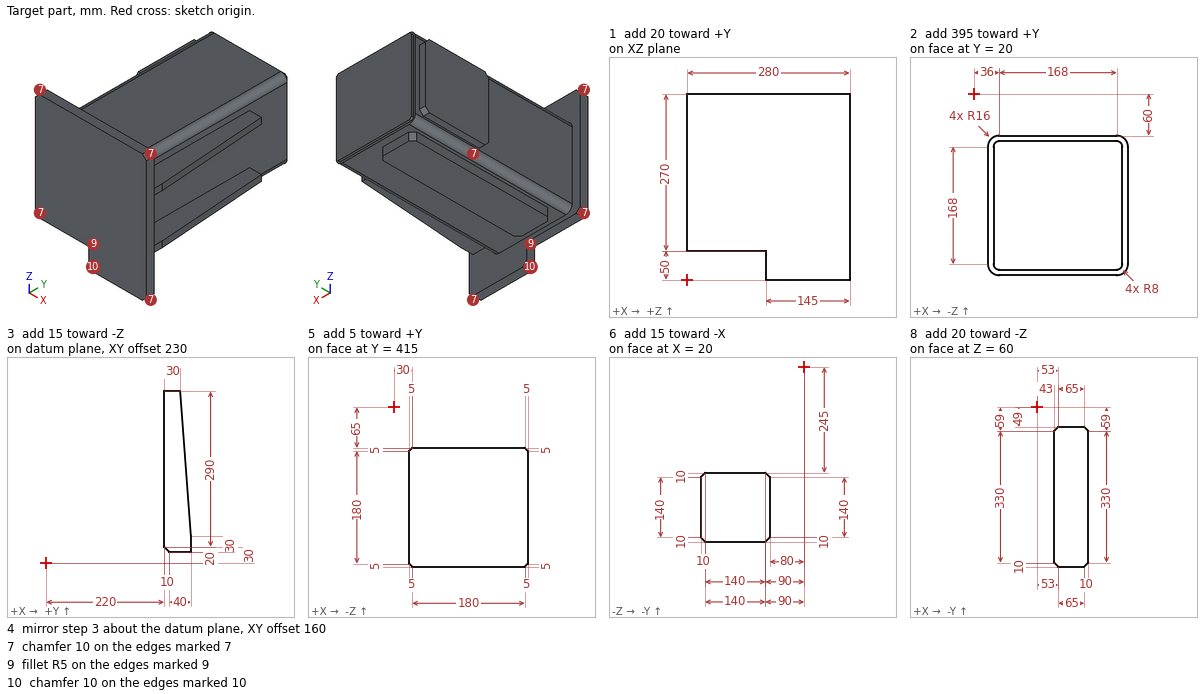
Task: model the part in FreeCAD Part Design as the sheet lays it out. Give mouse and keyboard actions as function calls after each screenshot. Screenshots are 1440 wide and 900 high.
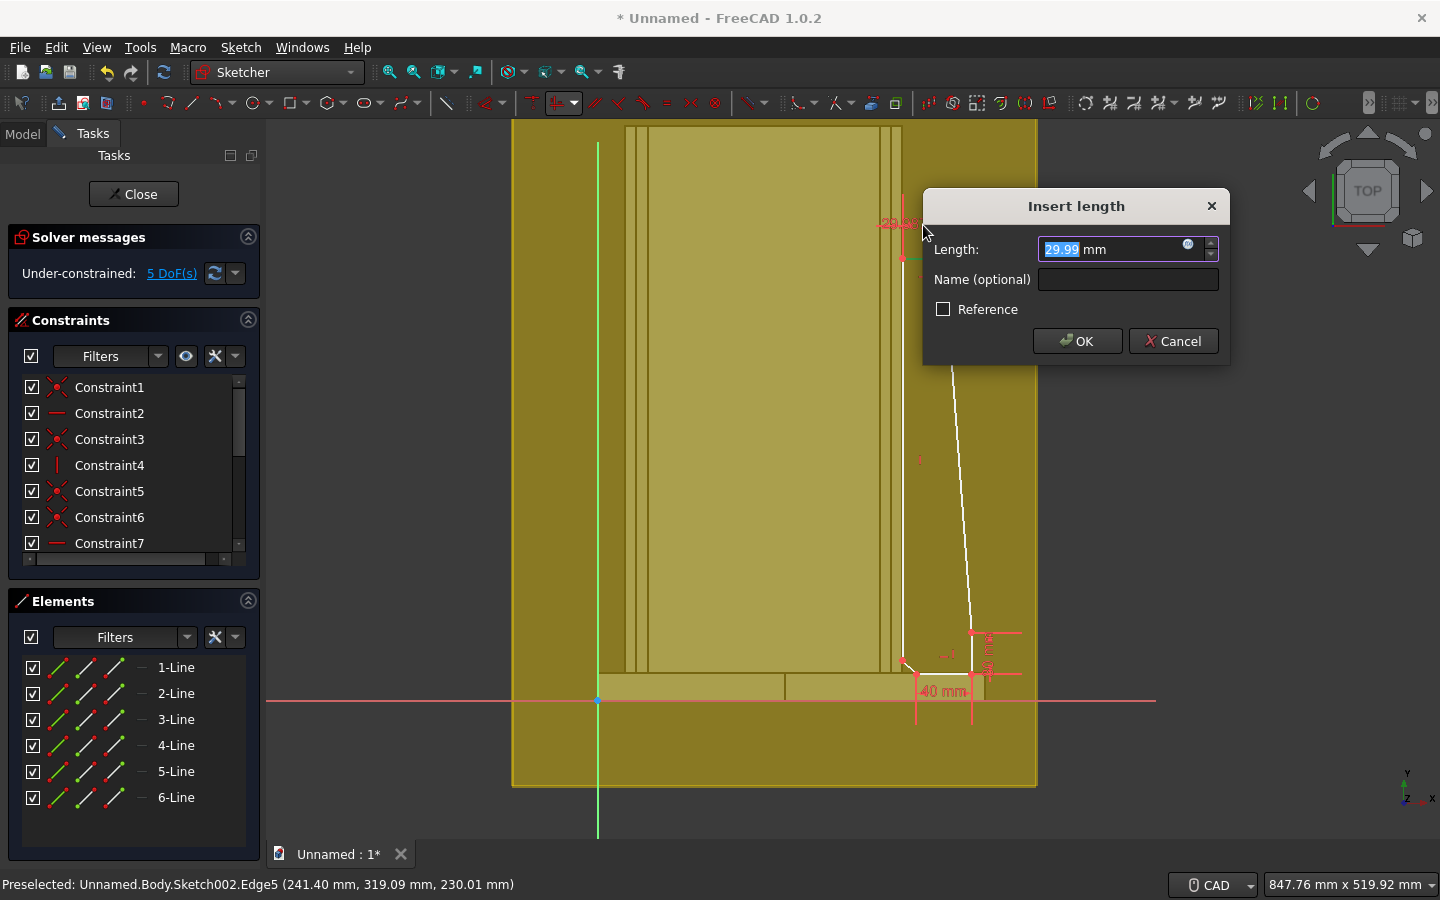
text(30)
key(Return)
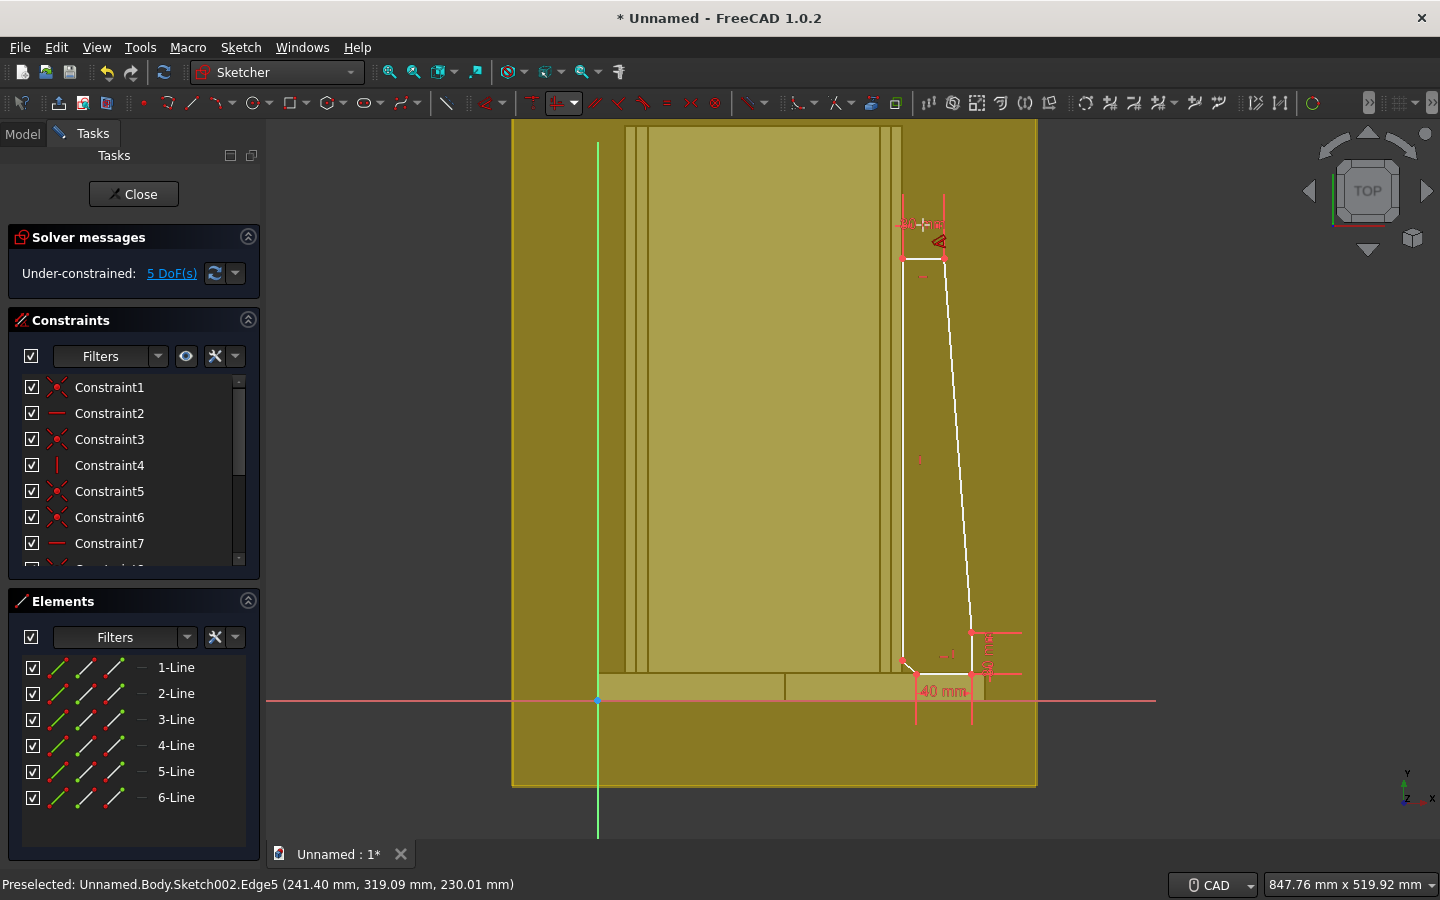
click(903, 379)
click(937, 460)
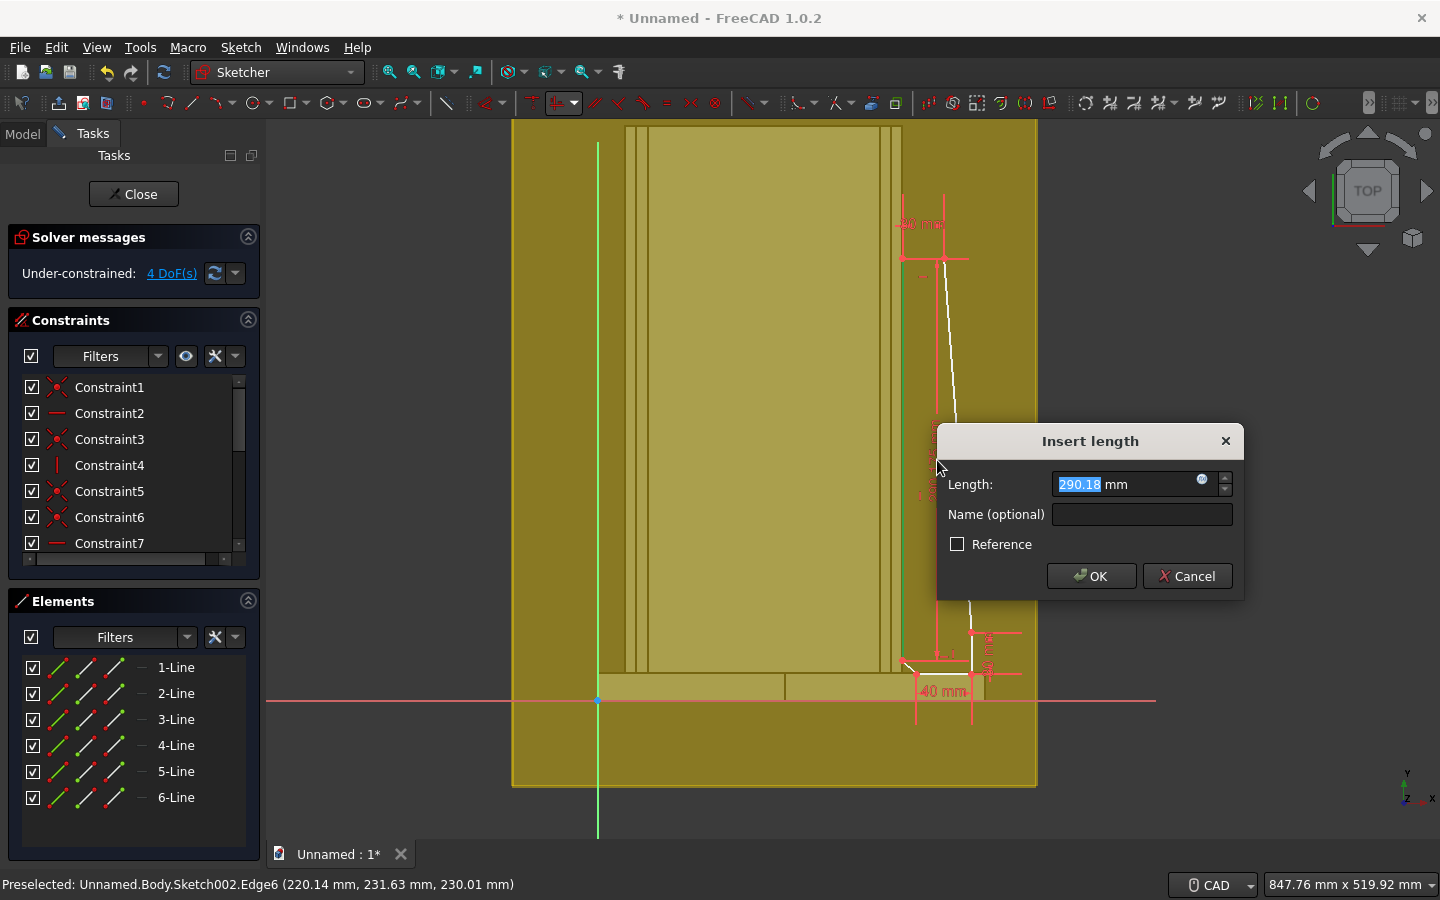
text(290)
key(Return)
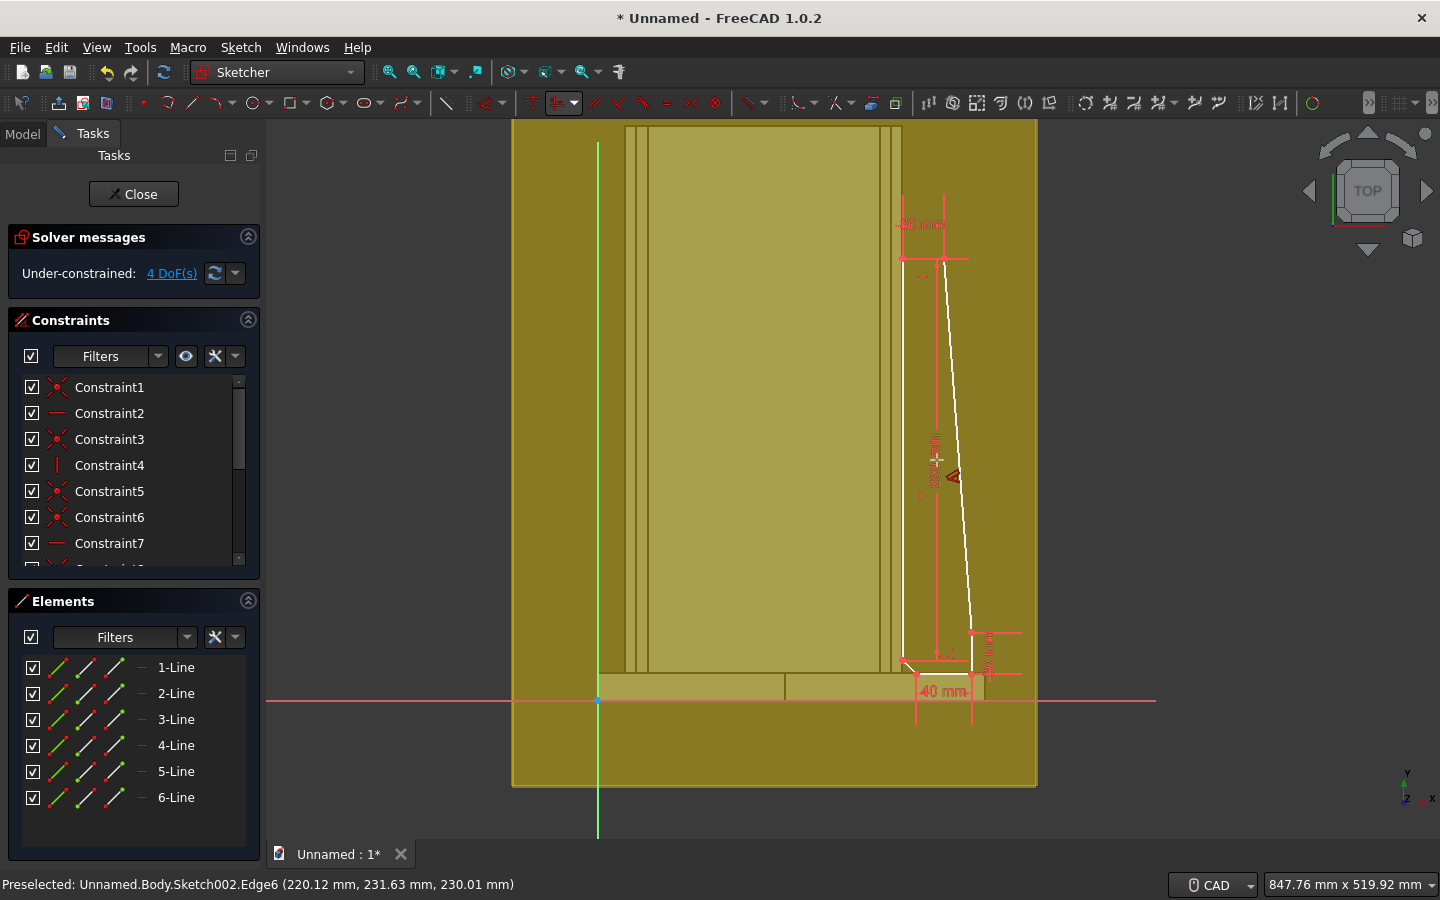
click(903, 661)
click(564, 681)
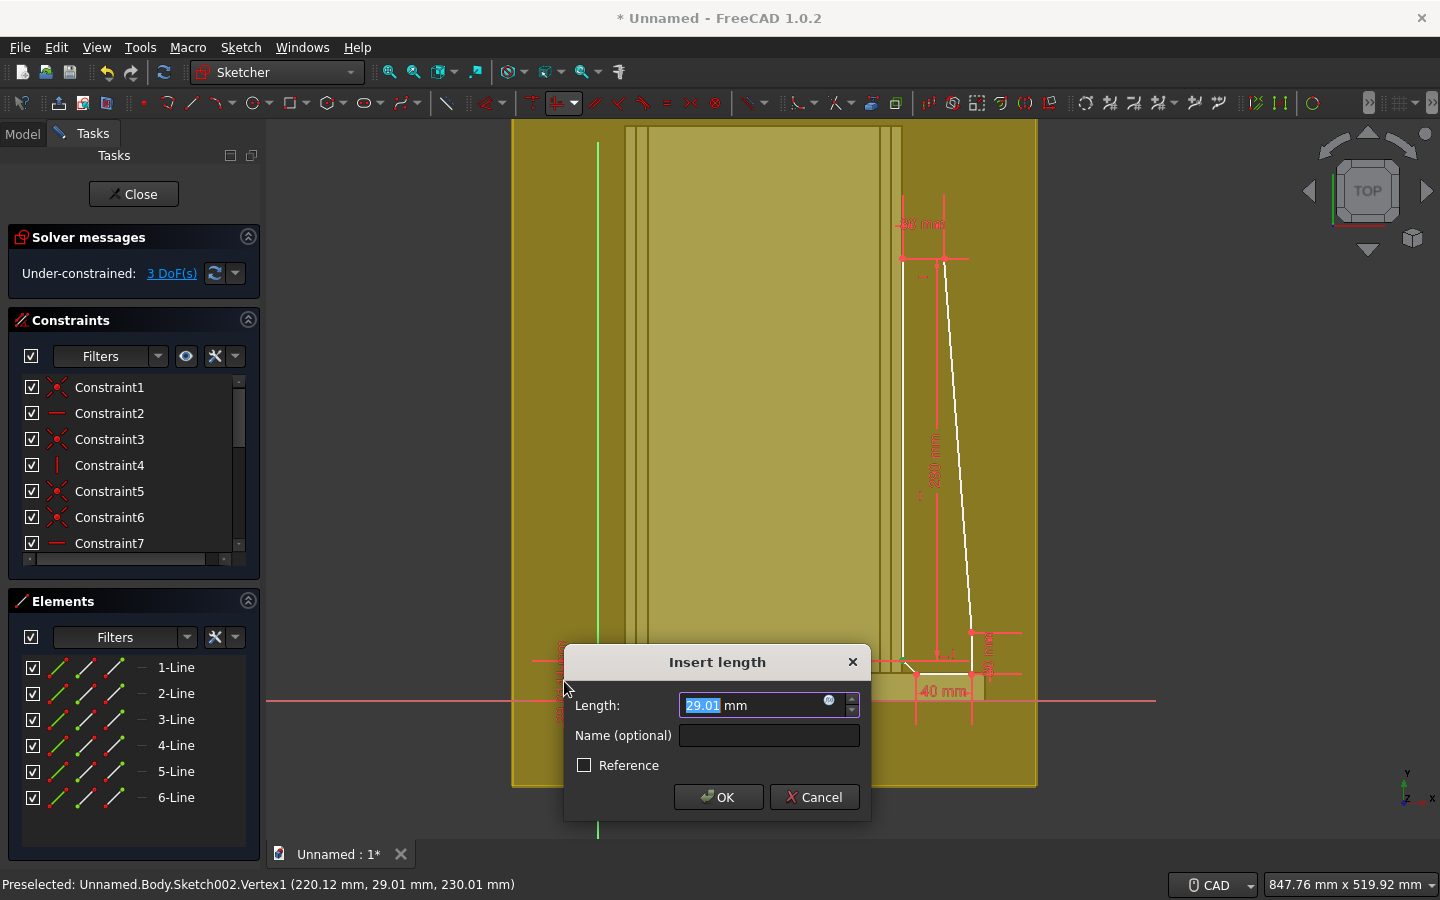
text(30)
key(Return)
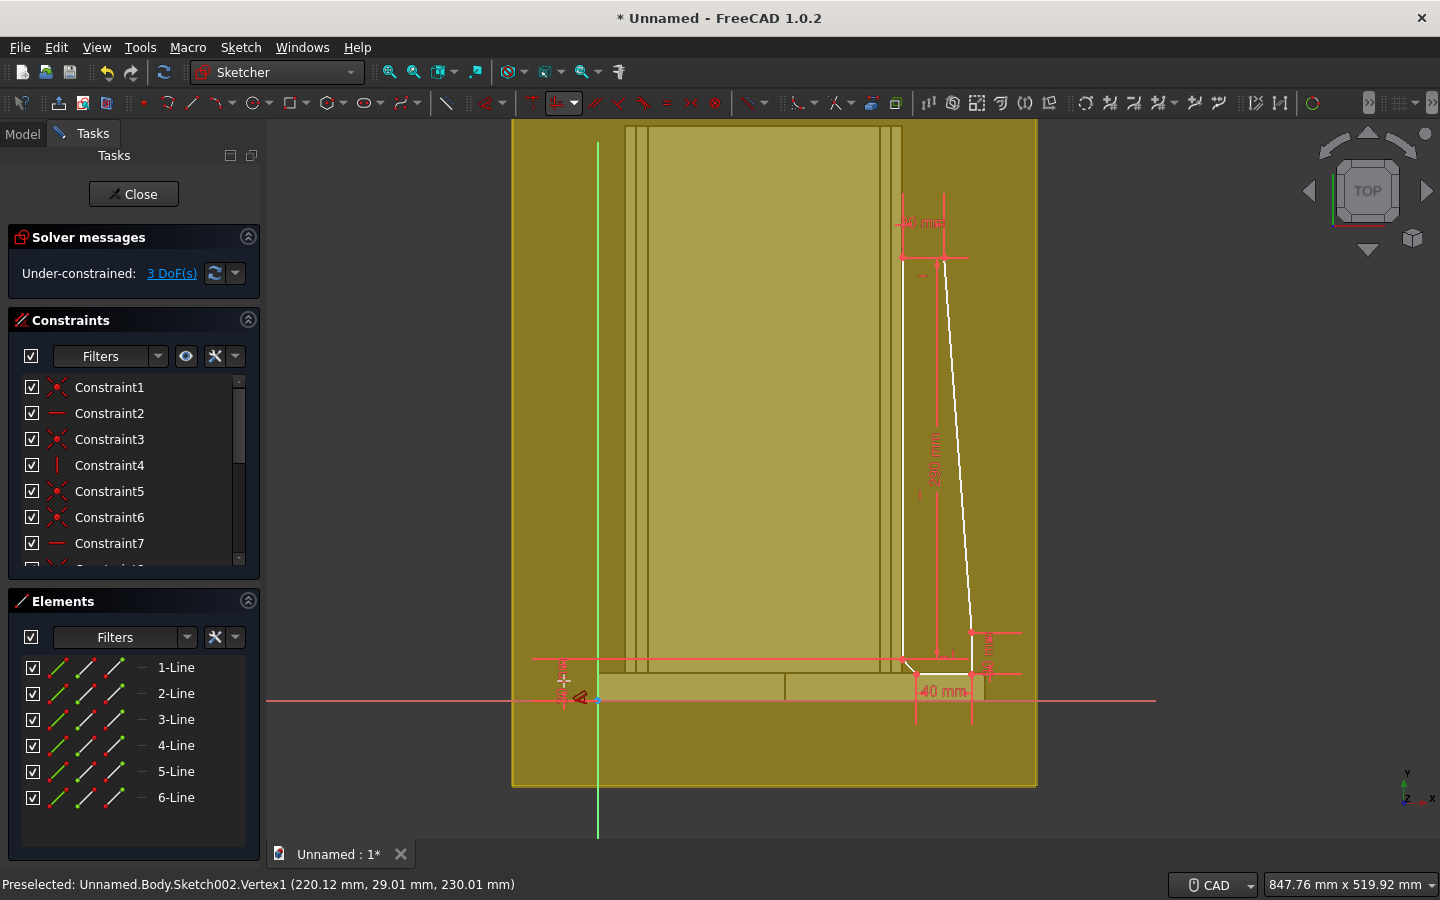
scroll(916, 674, up, 2)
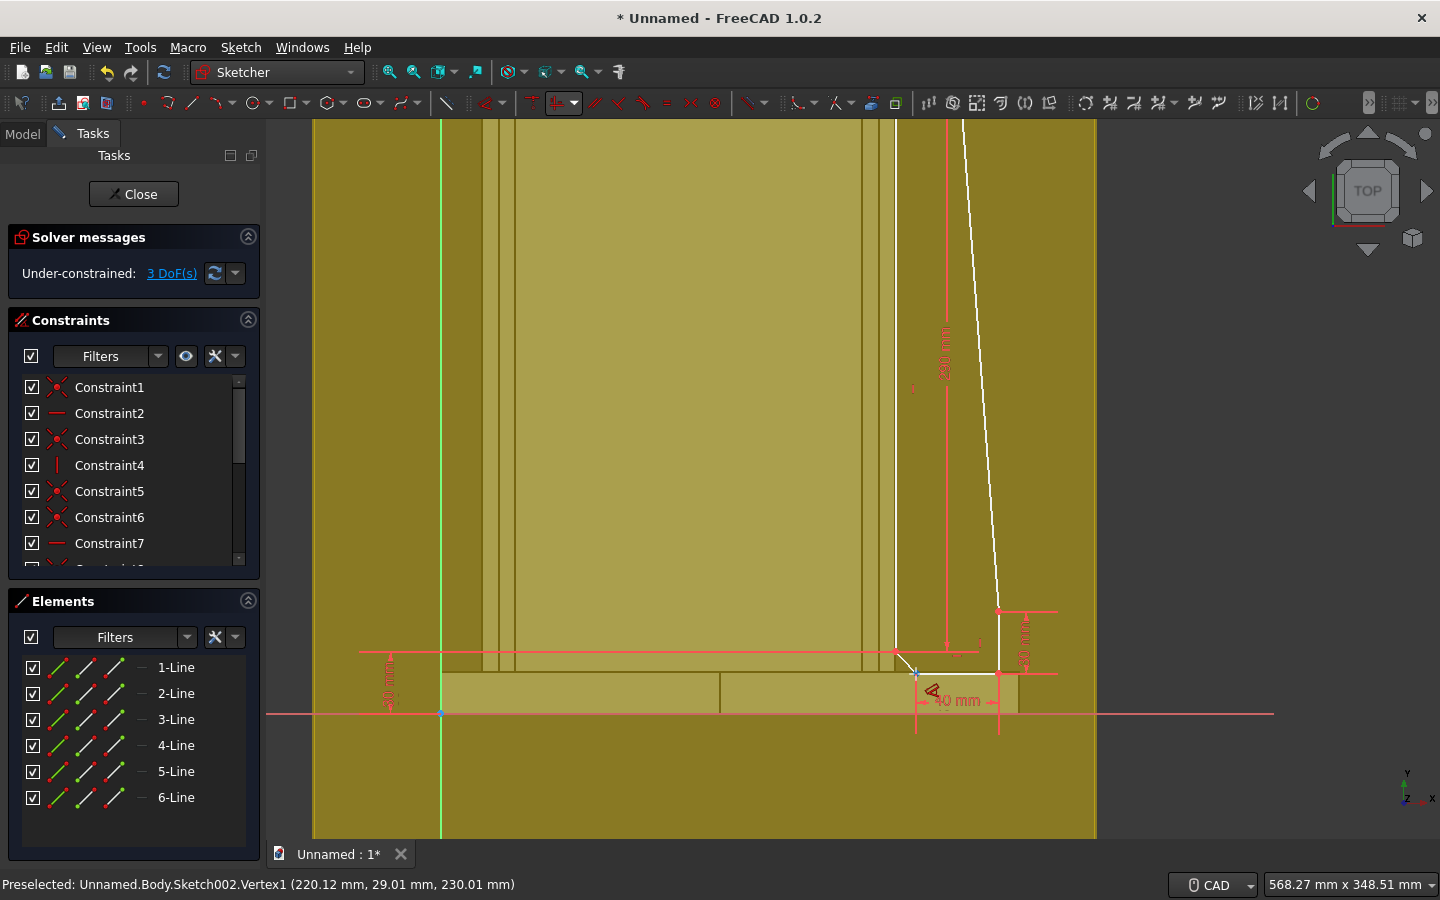
click(916, 674)
click(1022, 680)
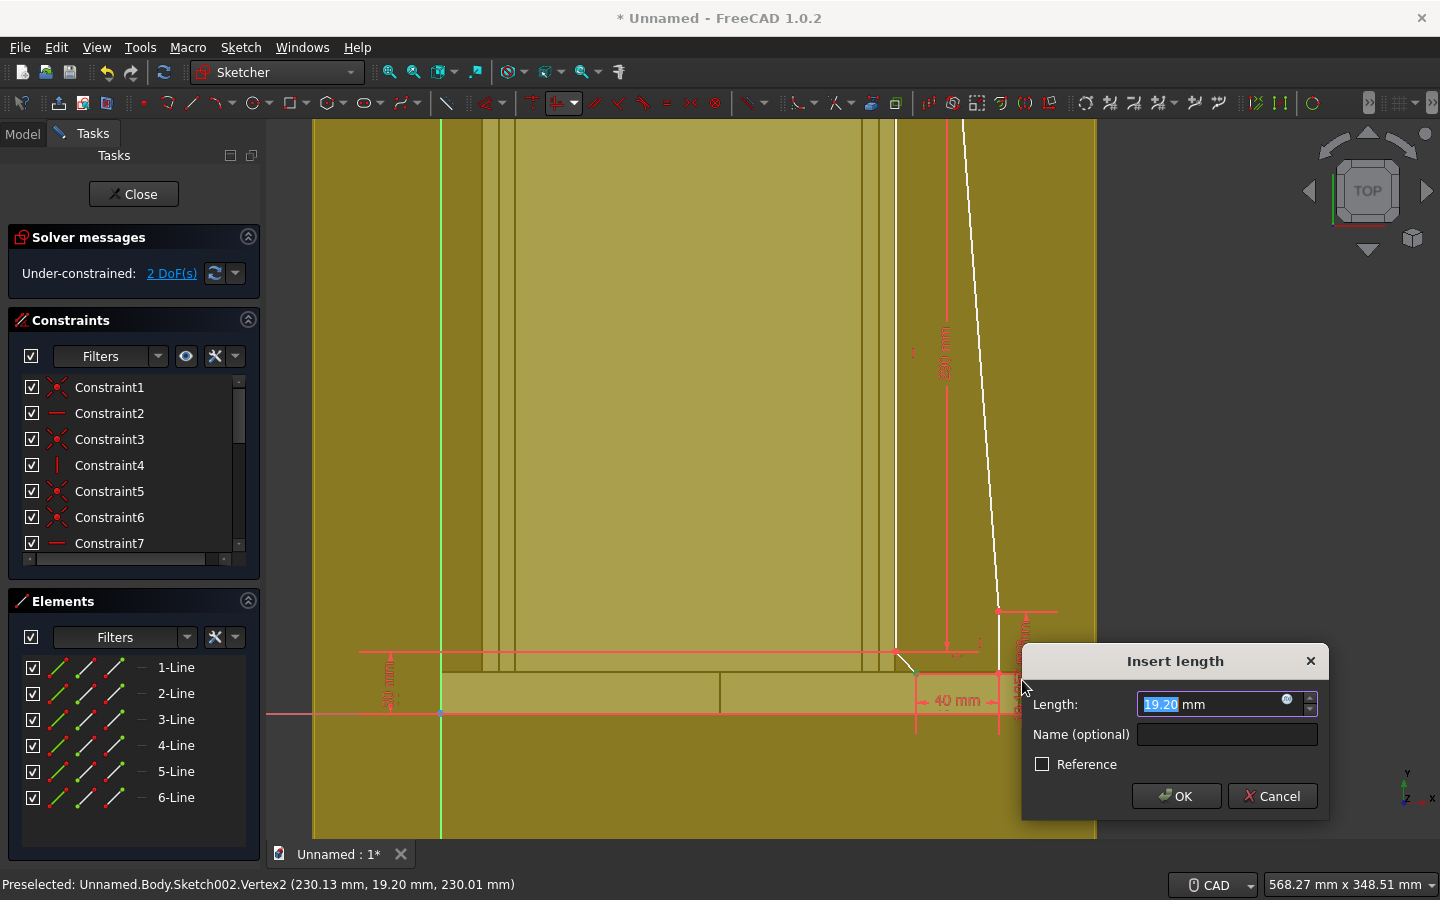
text(20)
key(Return)